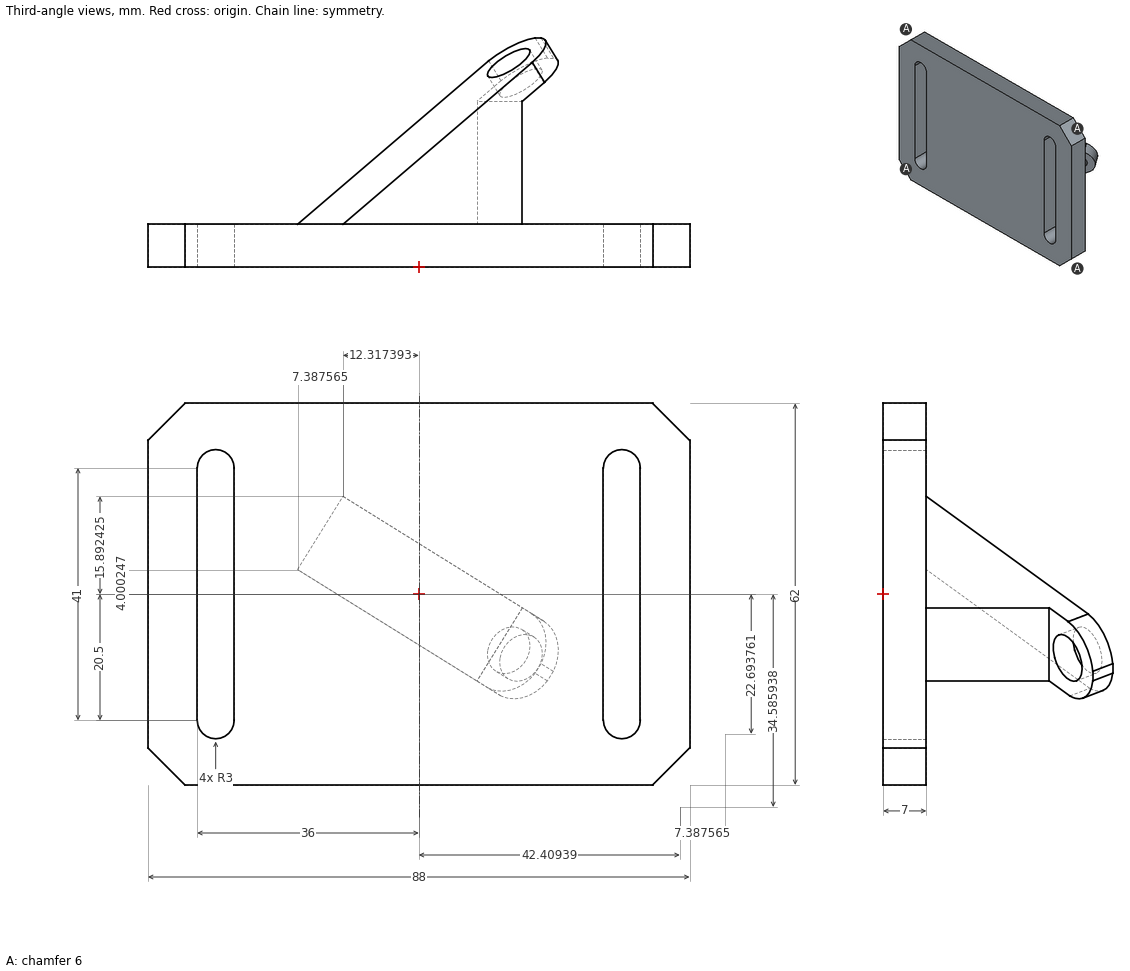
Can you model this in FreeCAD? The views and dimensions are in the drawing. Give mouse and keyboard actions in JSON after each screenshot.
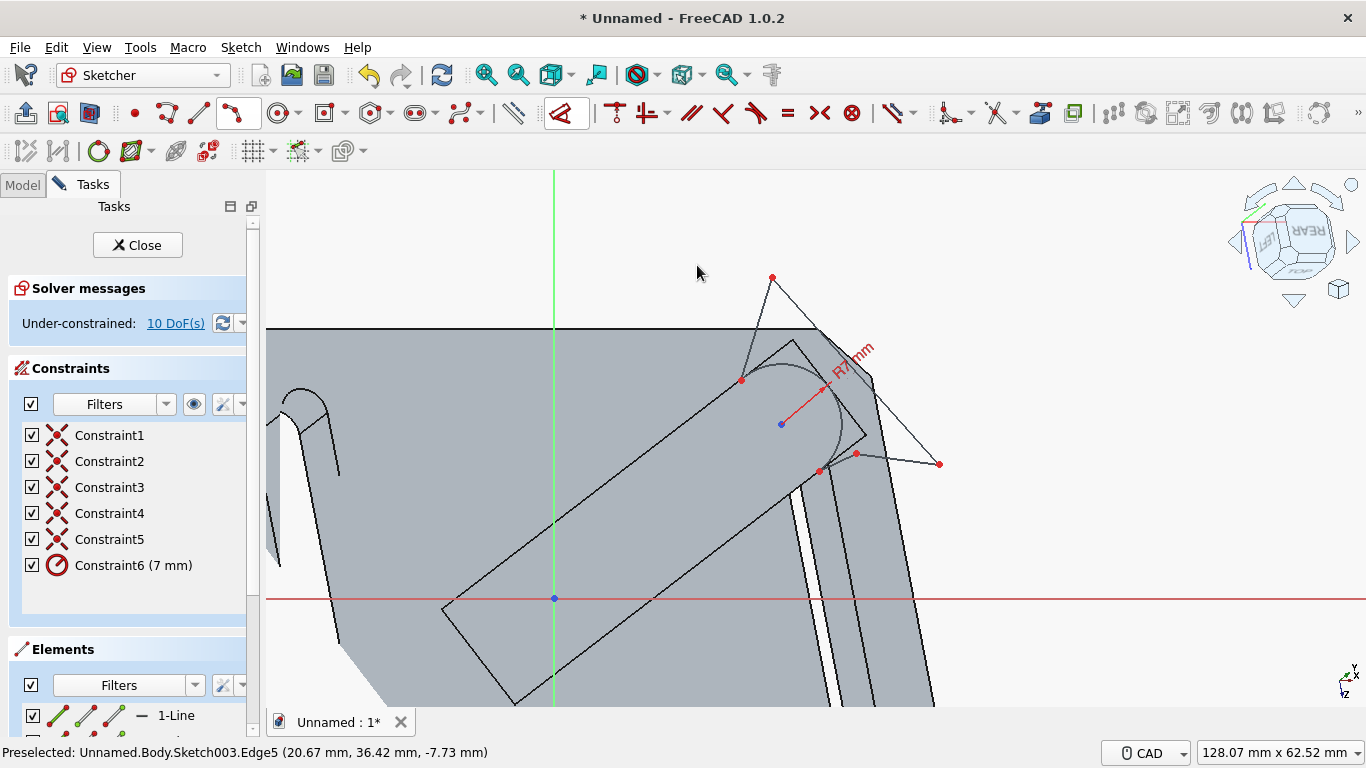
{"action": "left_click", "coordinate": [845, 459]}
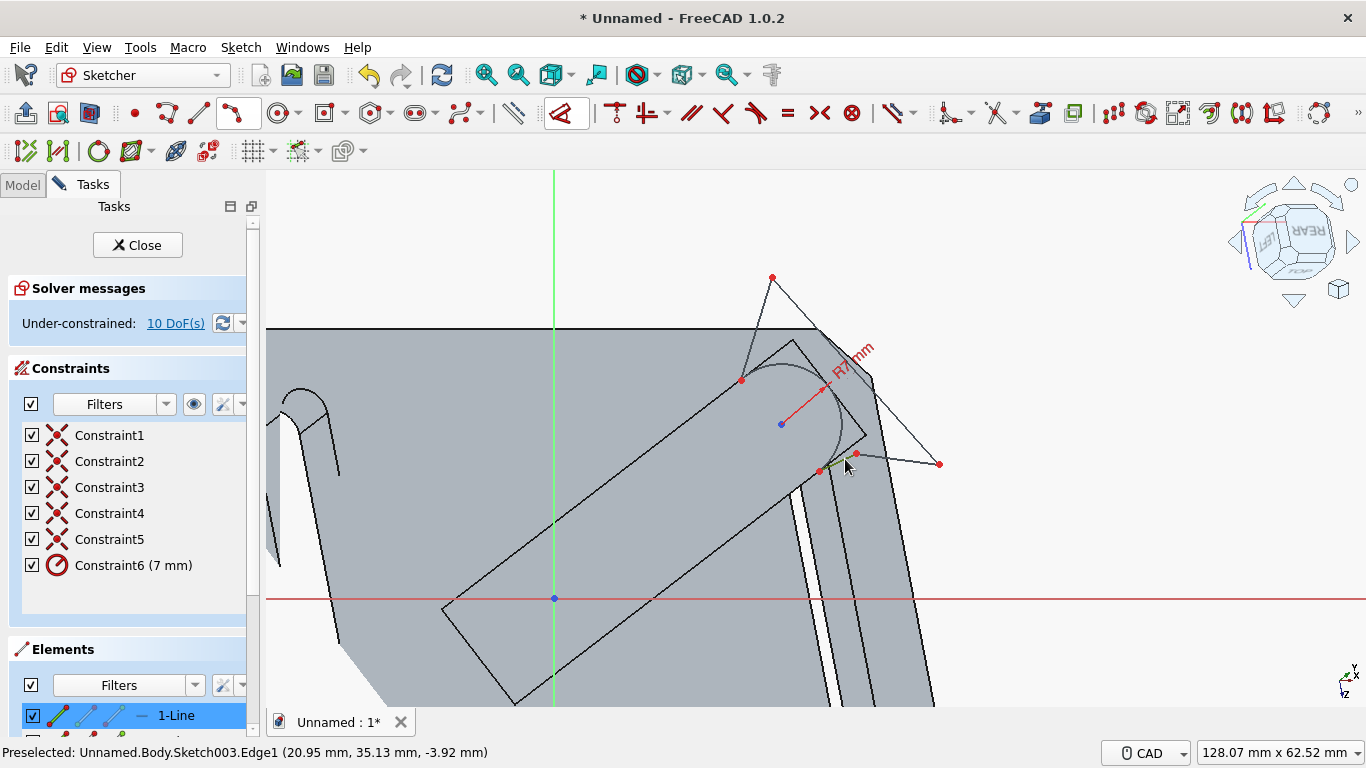
{"action": "key", "text": "l"}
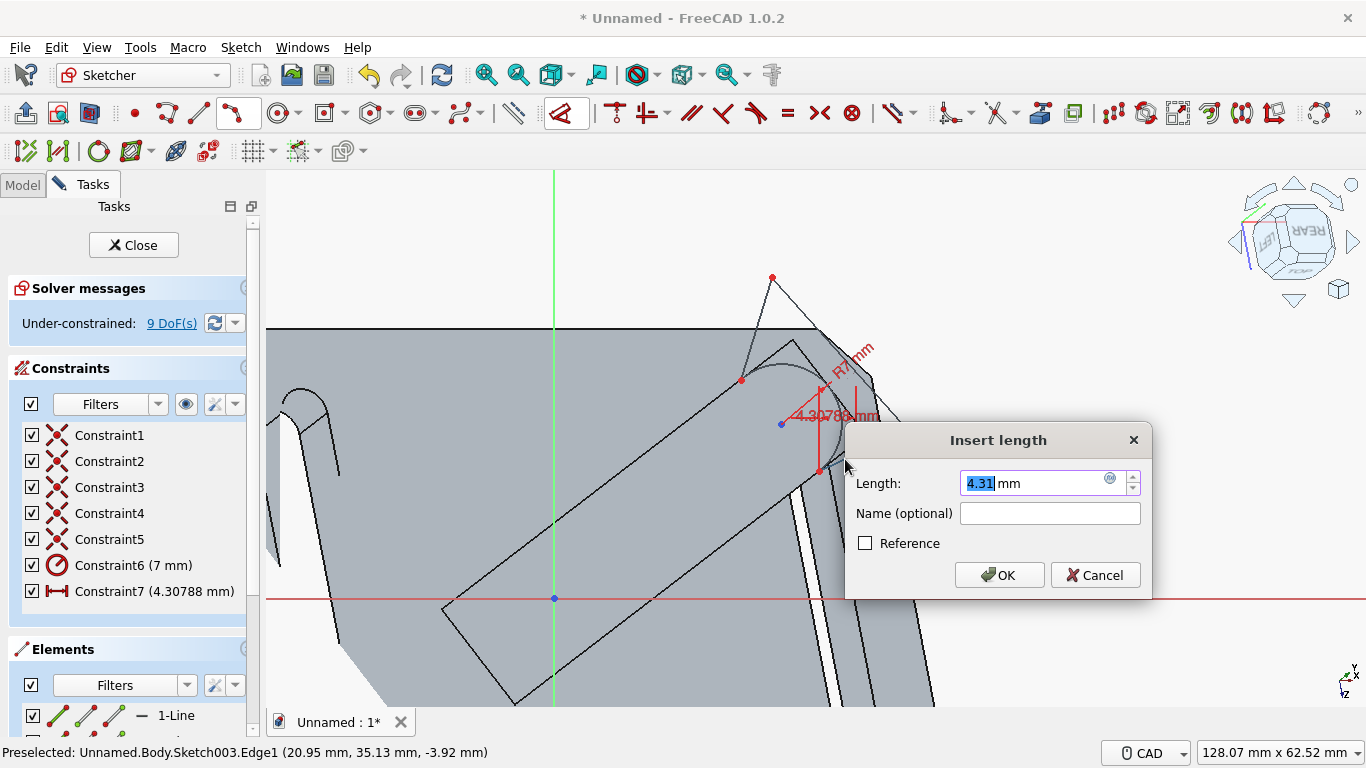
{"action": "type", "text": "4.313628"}
{"action": "key", "text": "Return"}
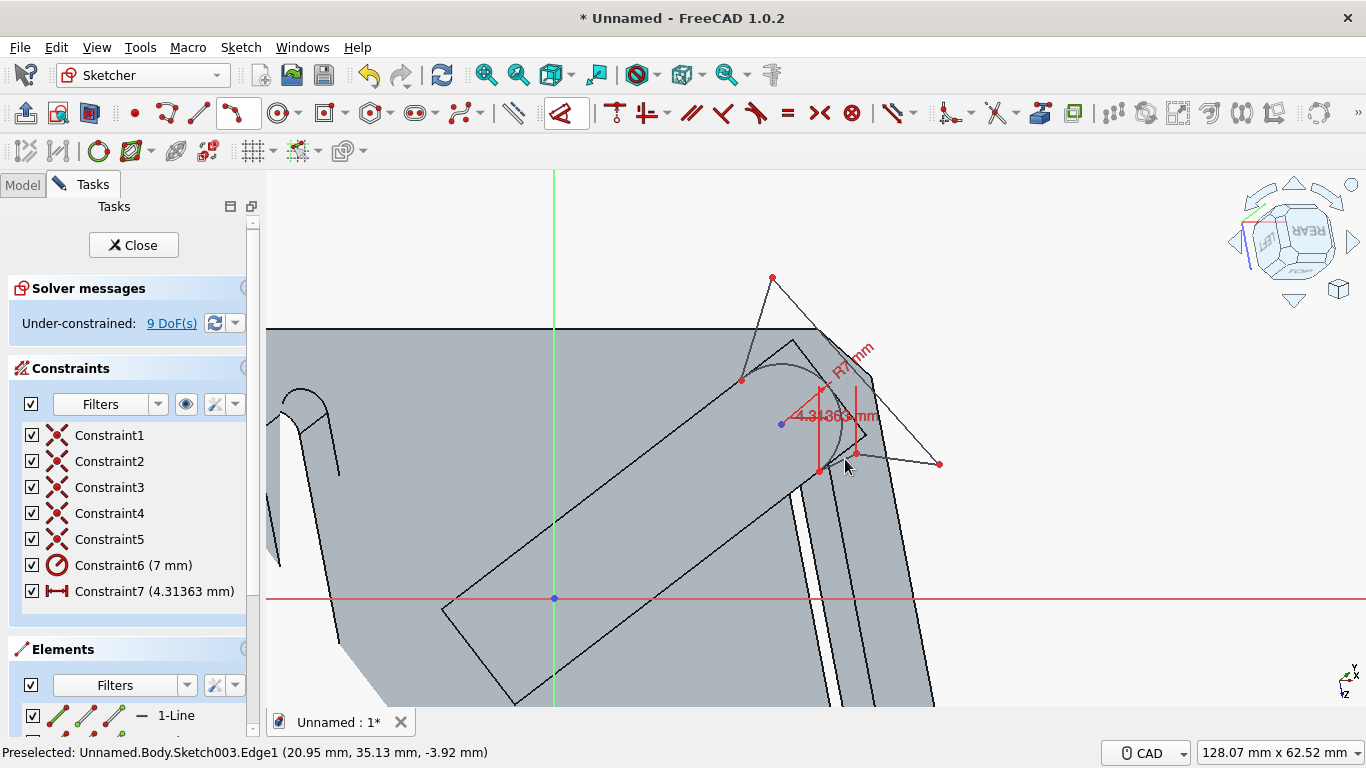
{"action": "scroll", "coordinate": [845, 459], "scroll_direction": "up", "scroll_amount": 5}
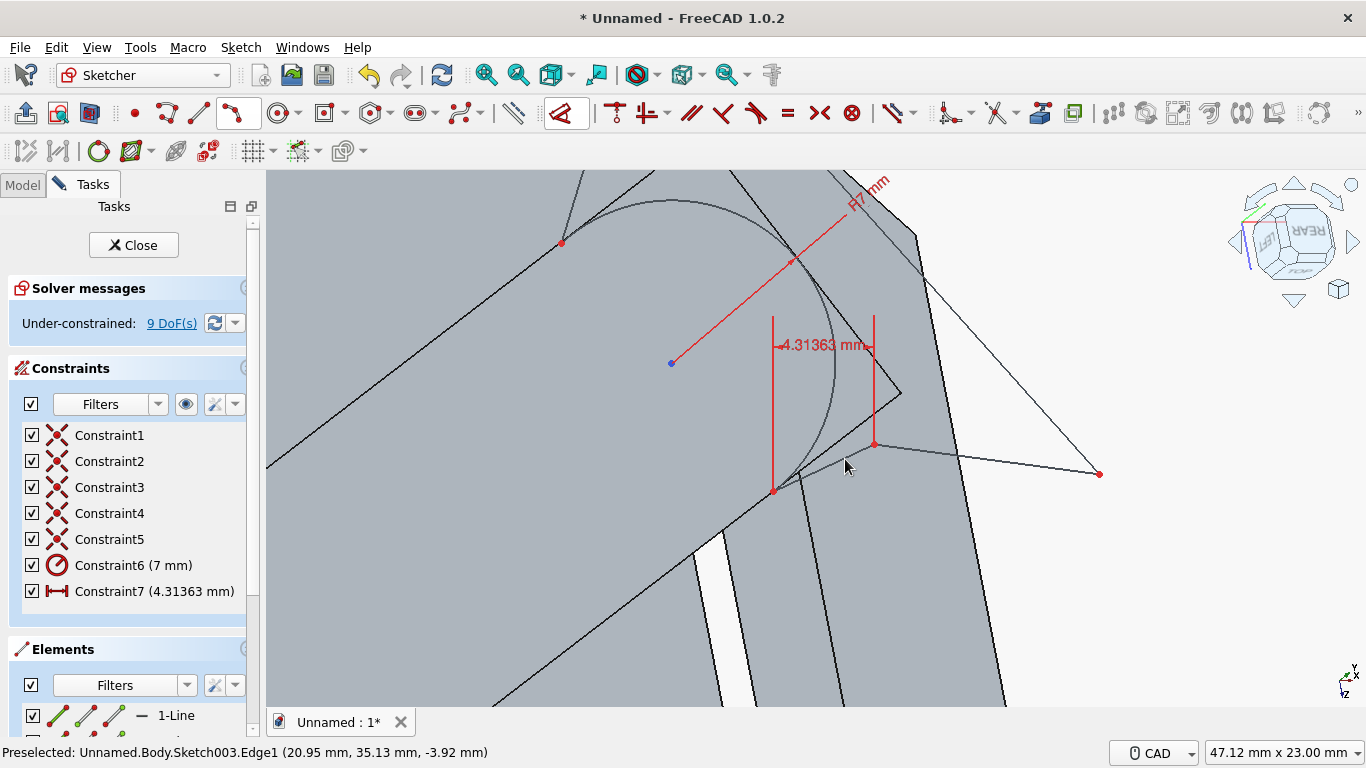
{"action": "left_click", "coordinate": [844, 459]}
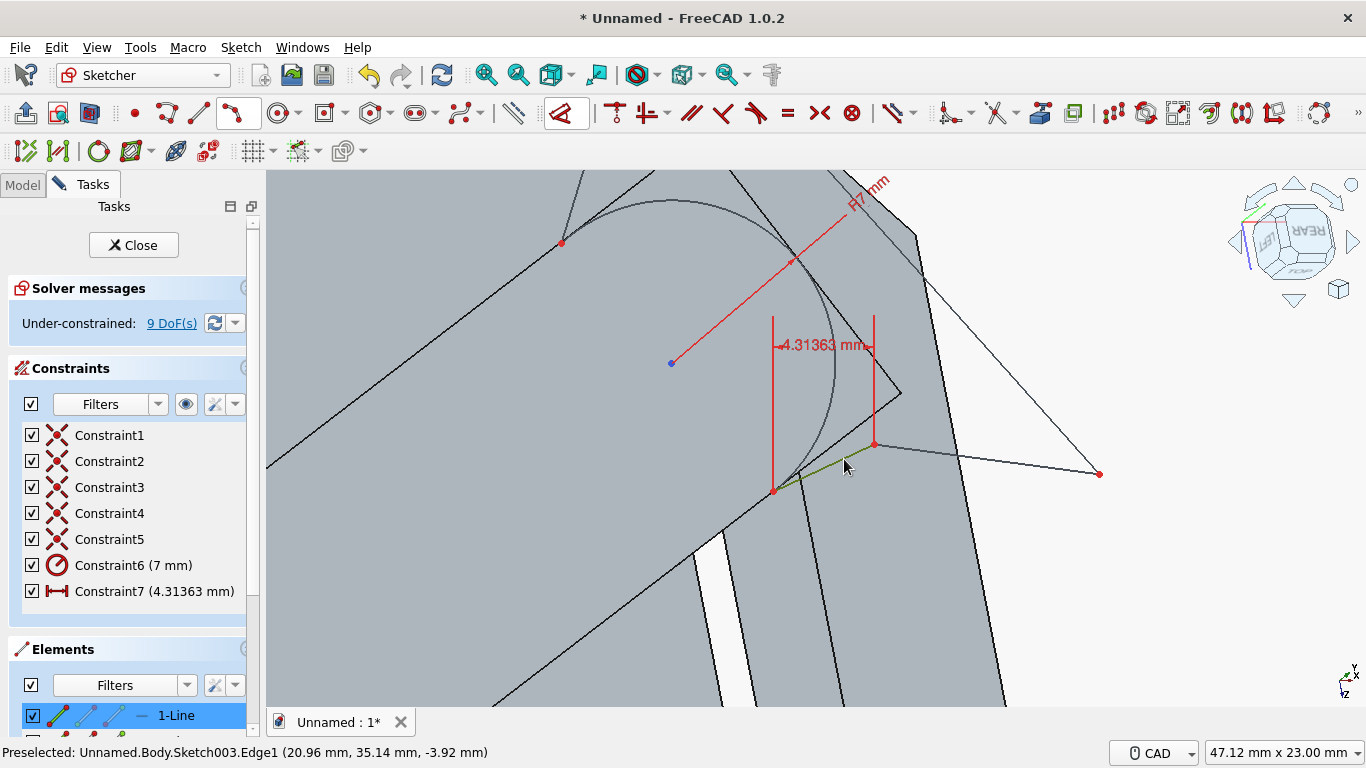
{"action": "key", "text": "i"}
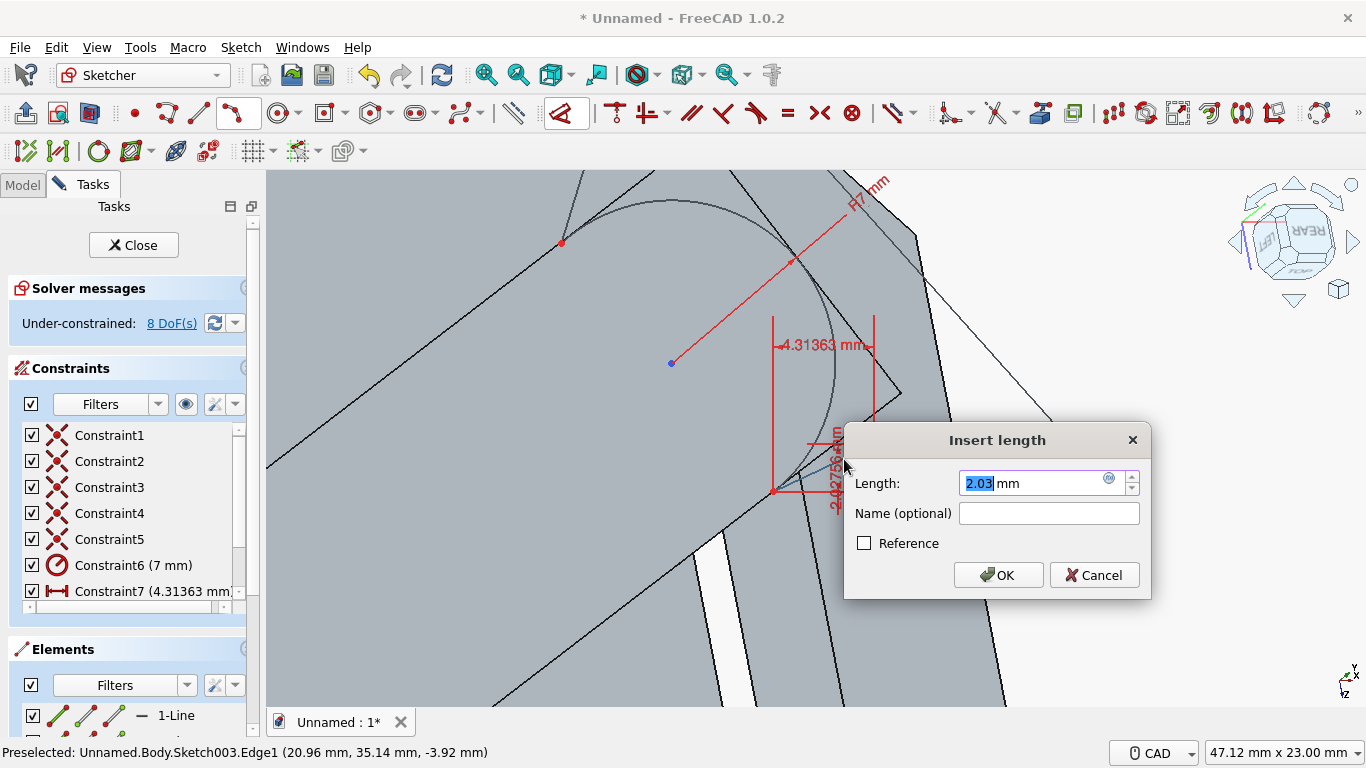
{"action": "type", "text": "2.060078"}
{"action": "key", "text": "Return"}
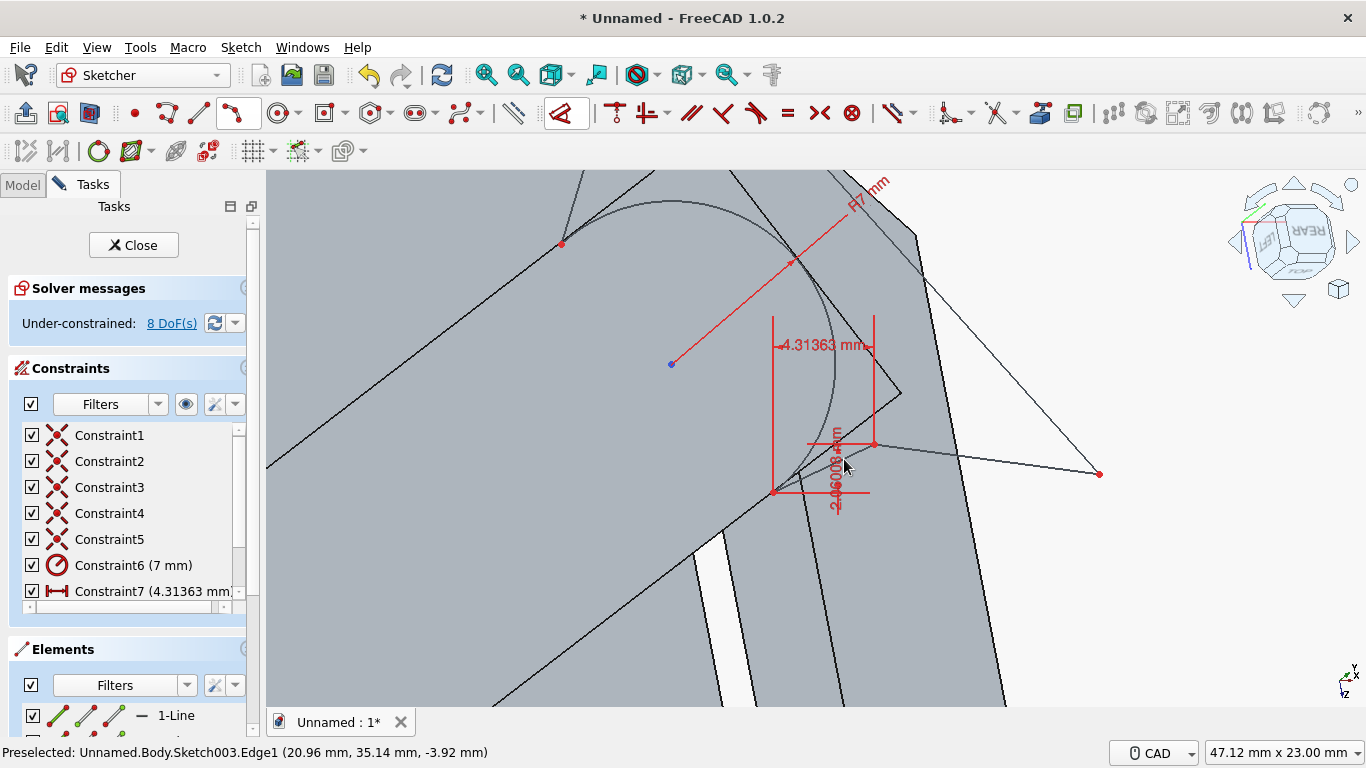
{"action": "left_click", "coordinate": [942, 453]}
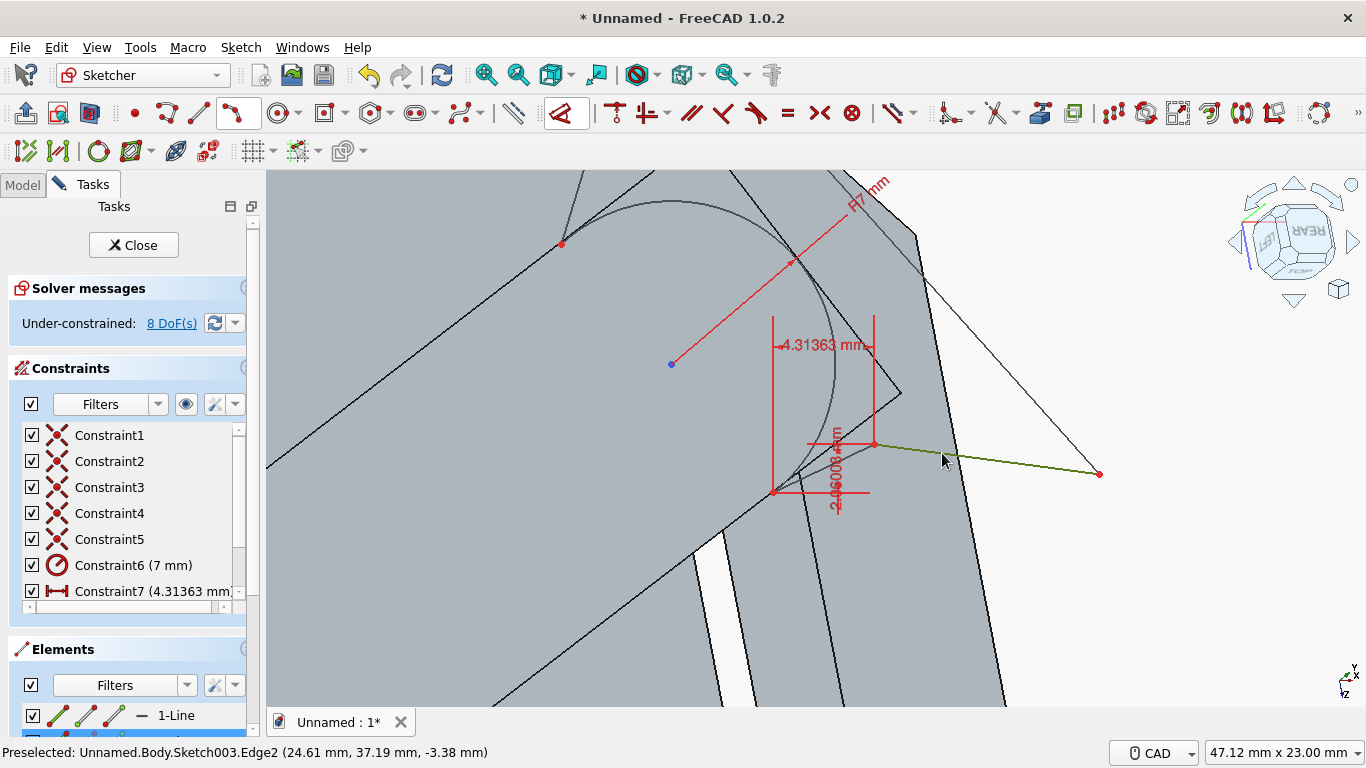
{"action": "left_click", "coordinate": [584, 114]}